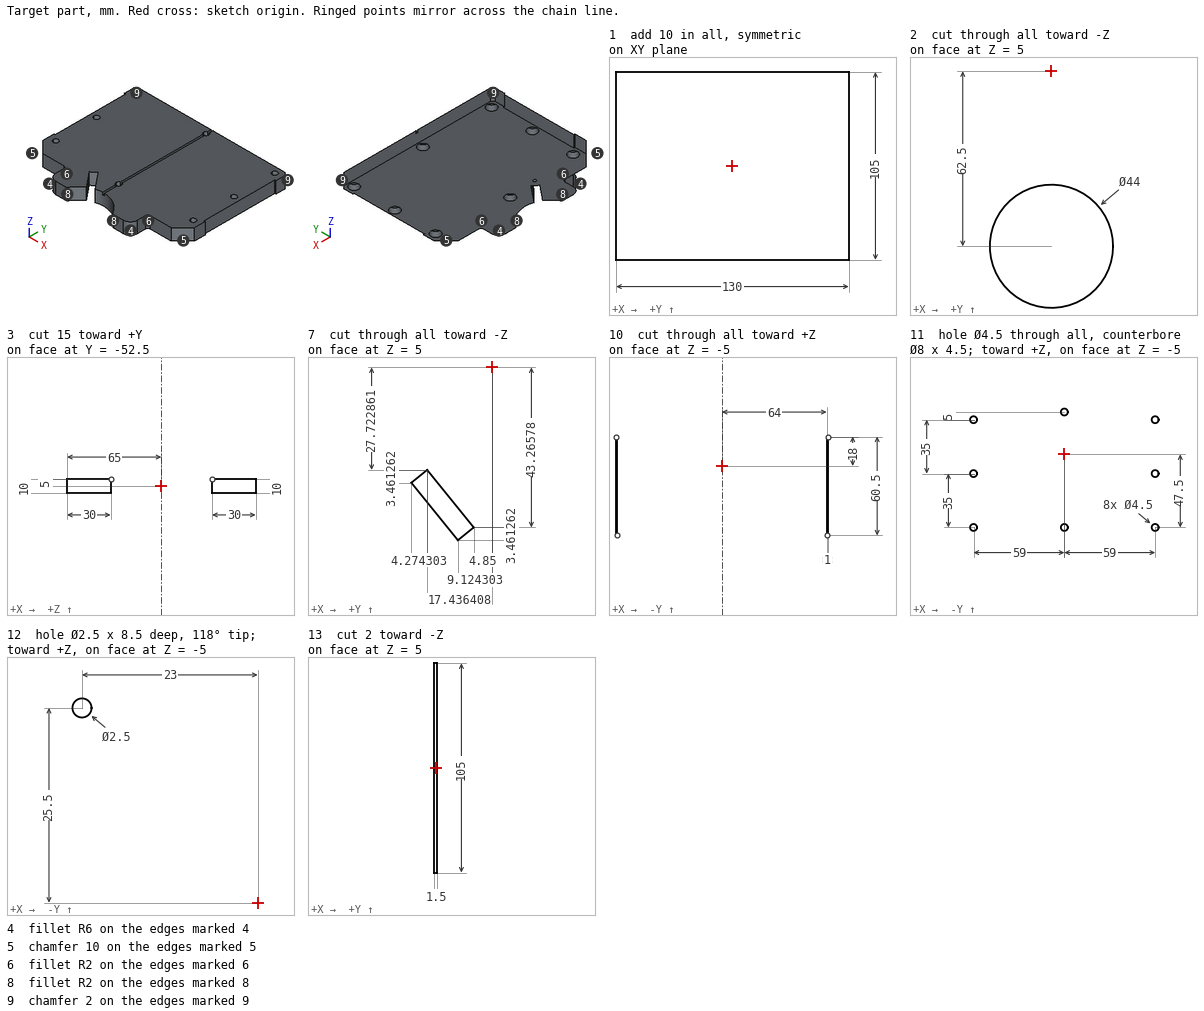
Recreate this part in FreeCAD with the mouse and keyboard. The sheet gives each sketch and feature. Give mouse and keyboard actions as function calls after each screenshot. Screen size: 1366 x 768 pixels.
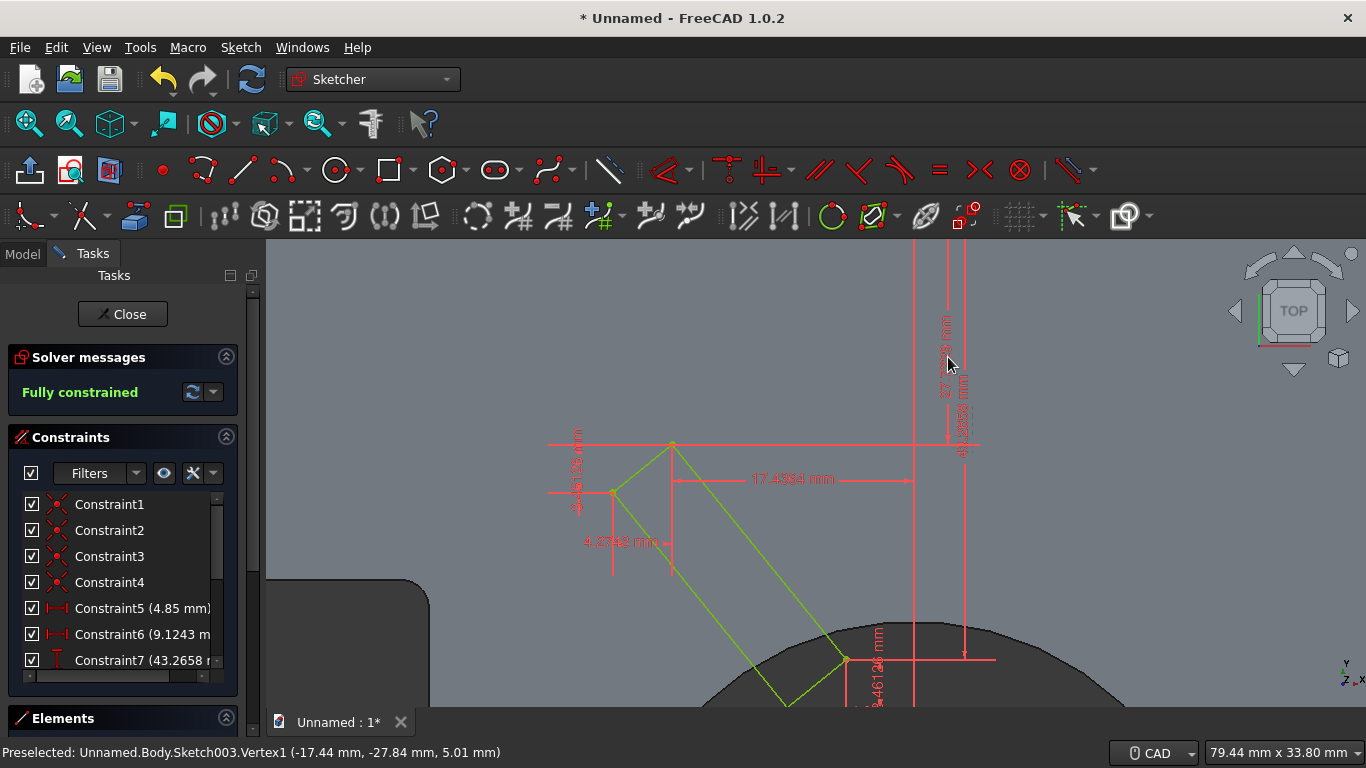
click(123, 314)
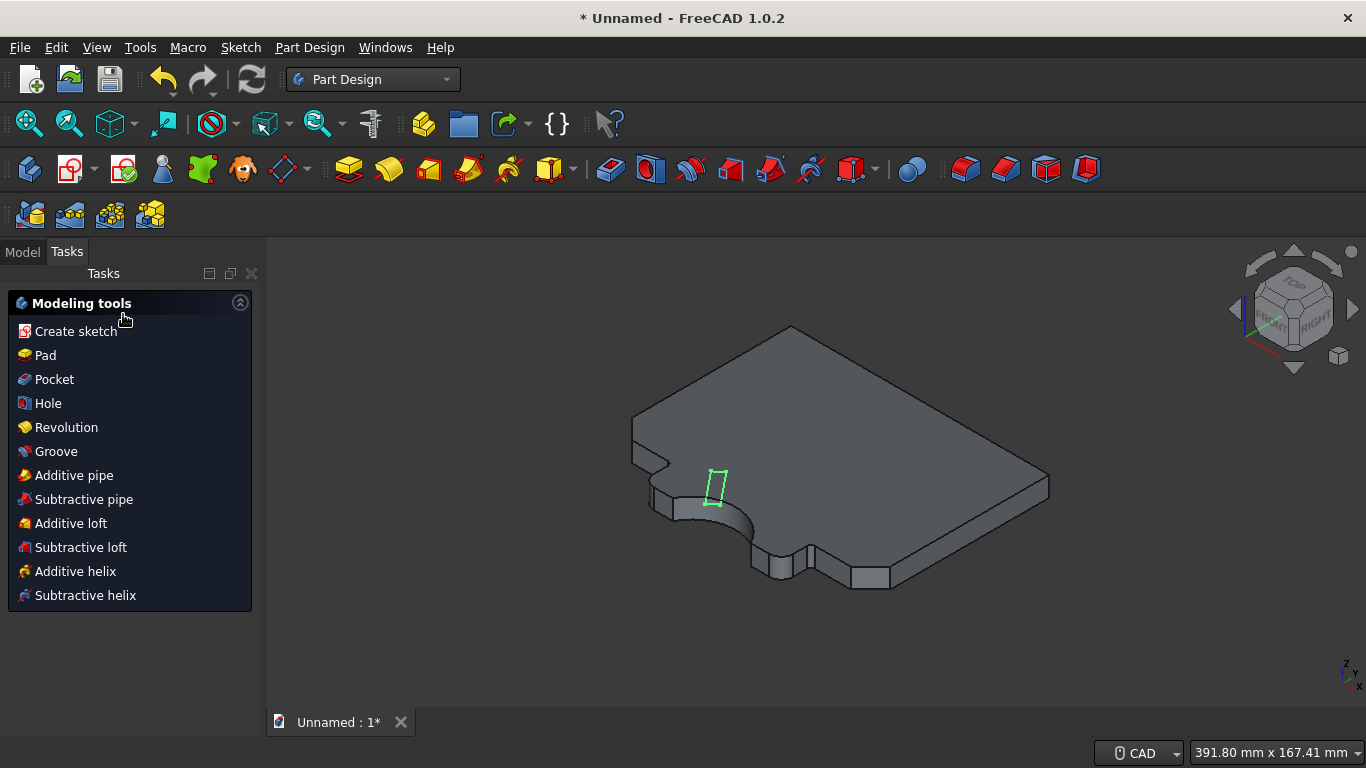
click(612, 170)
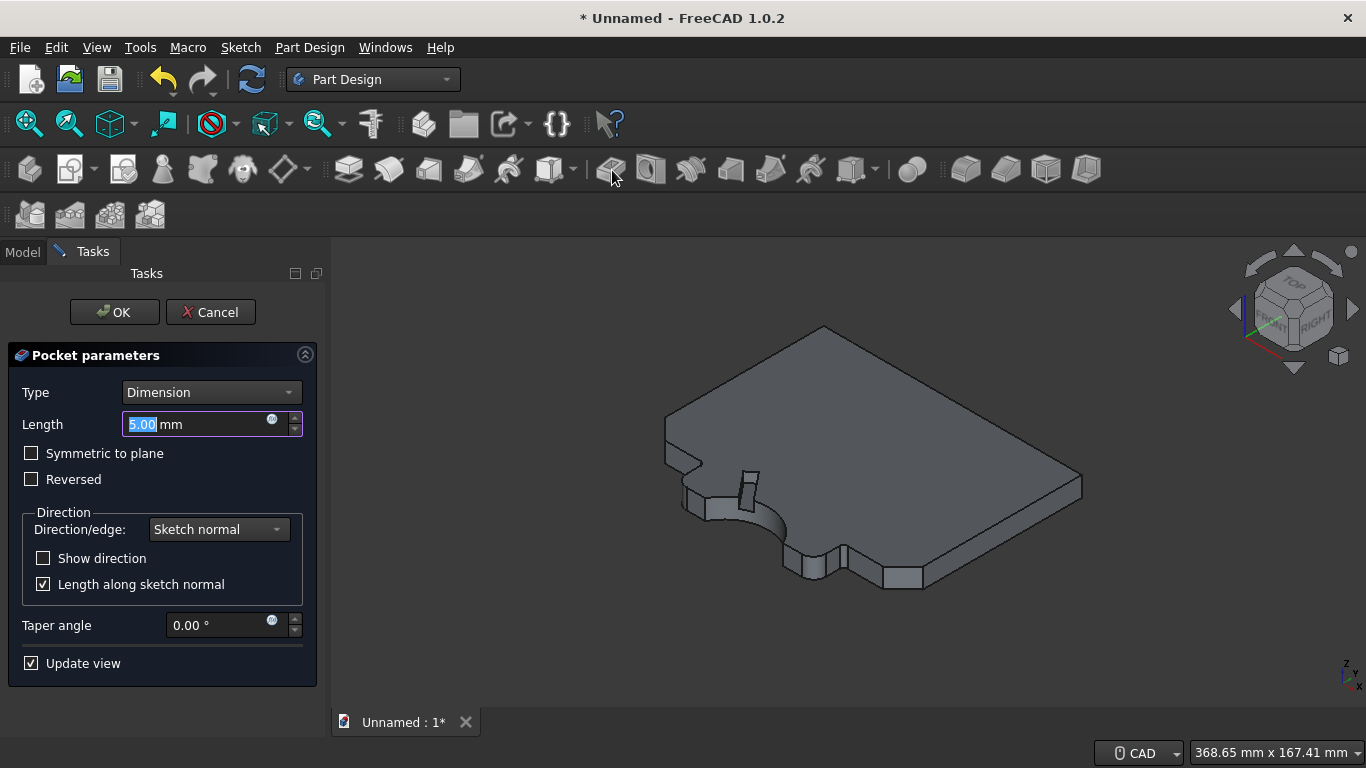
click(212, 392)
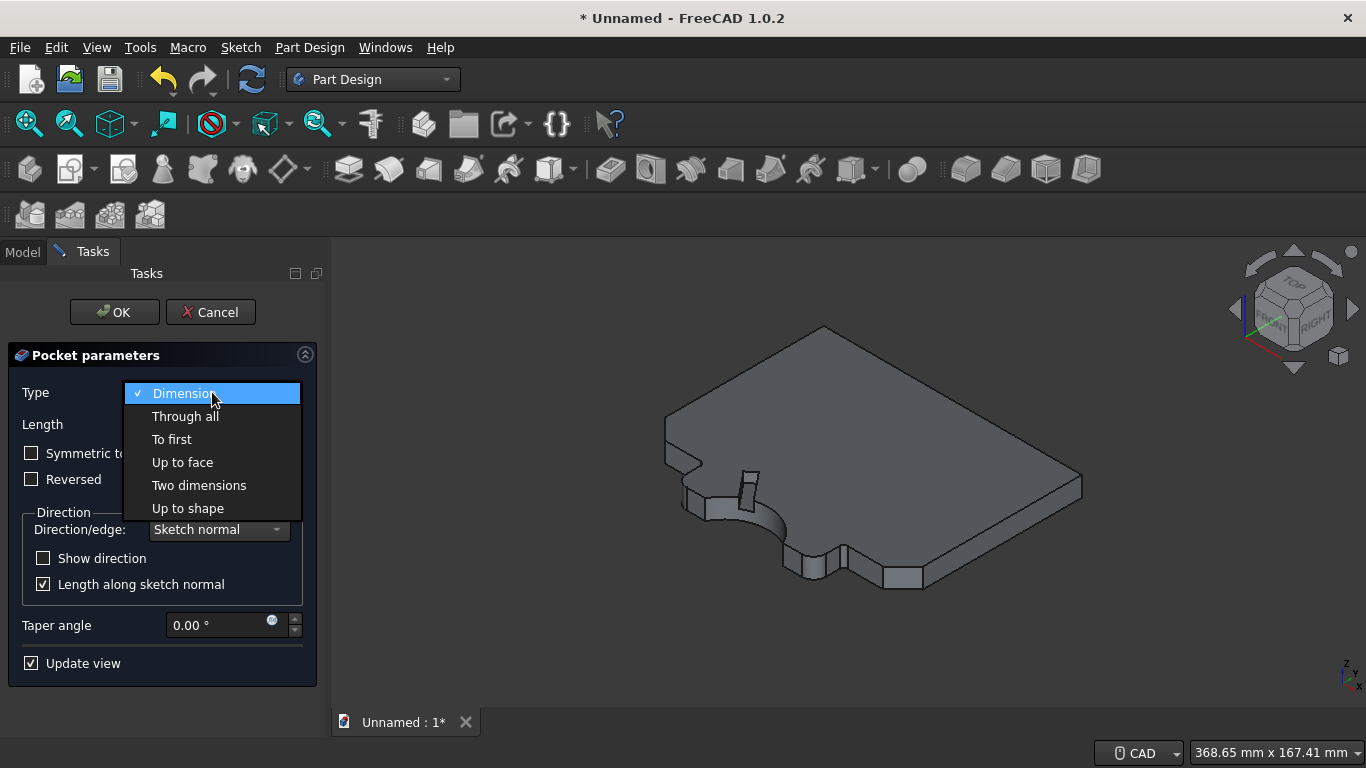
click(212, 416)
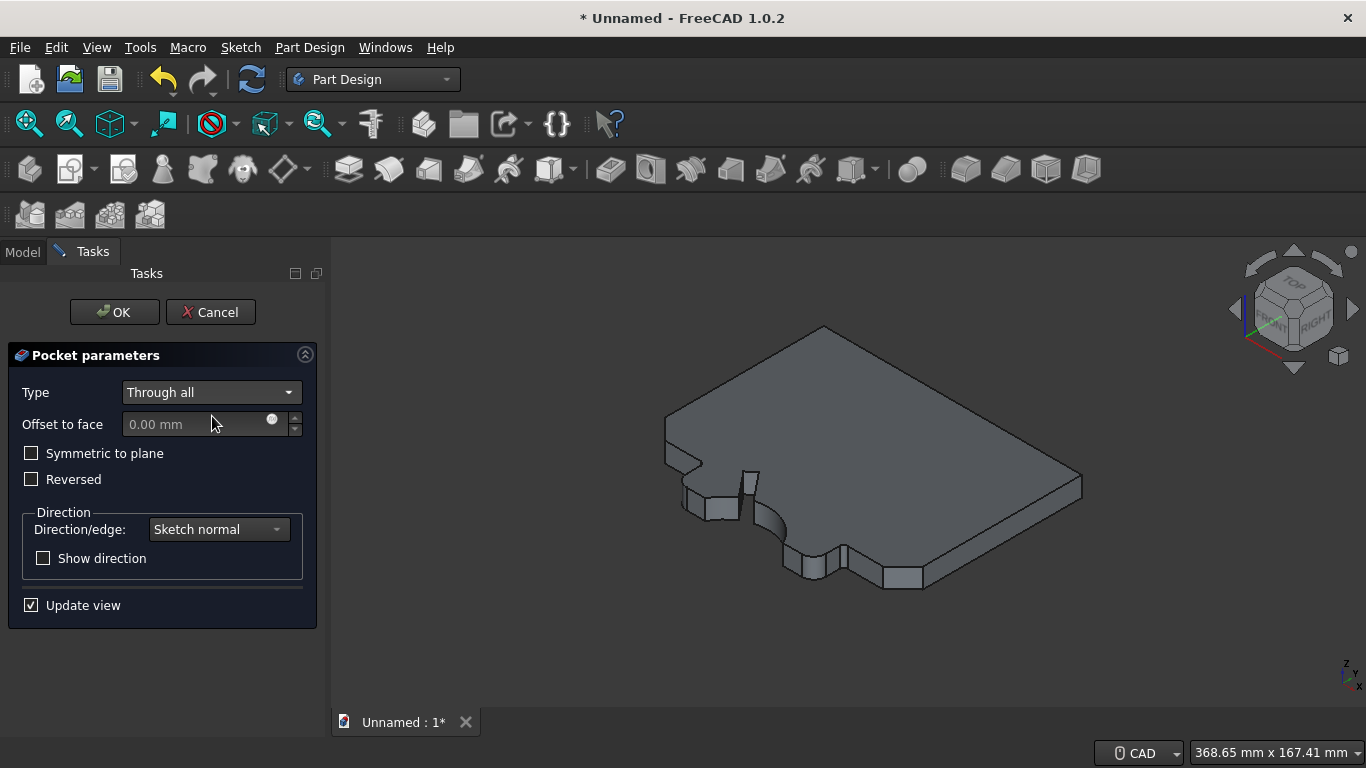
click(115, 312)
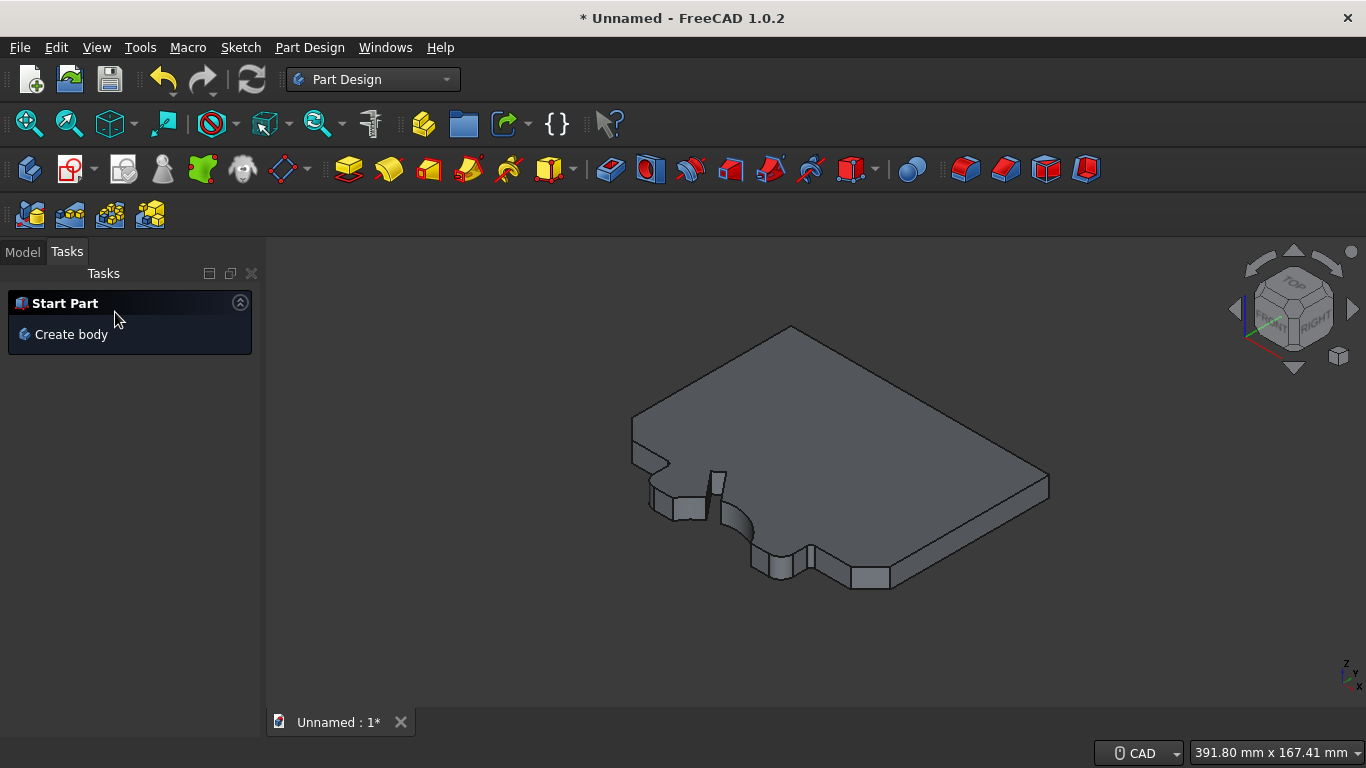
click(673, 509)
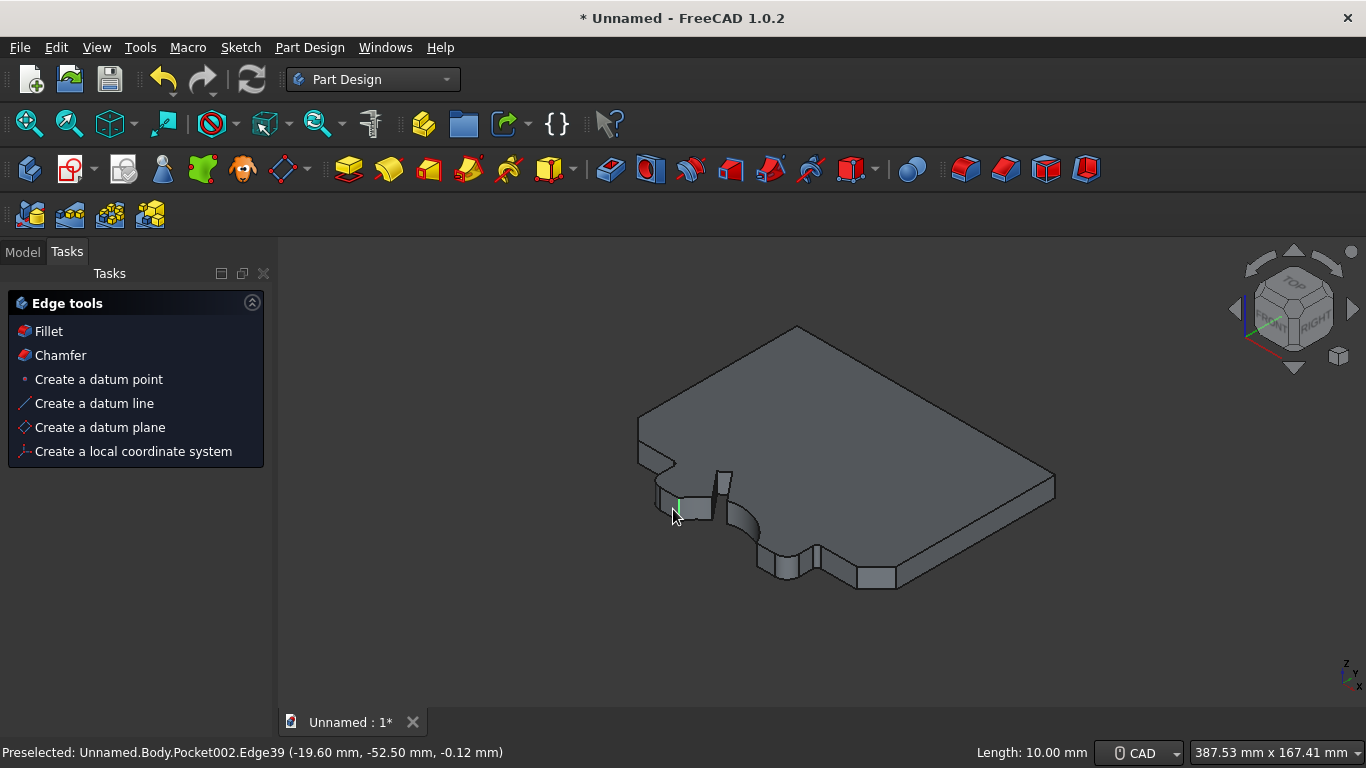
key(2)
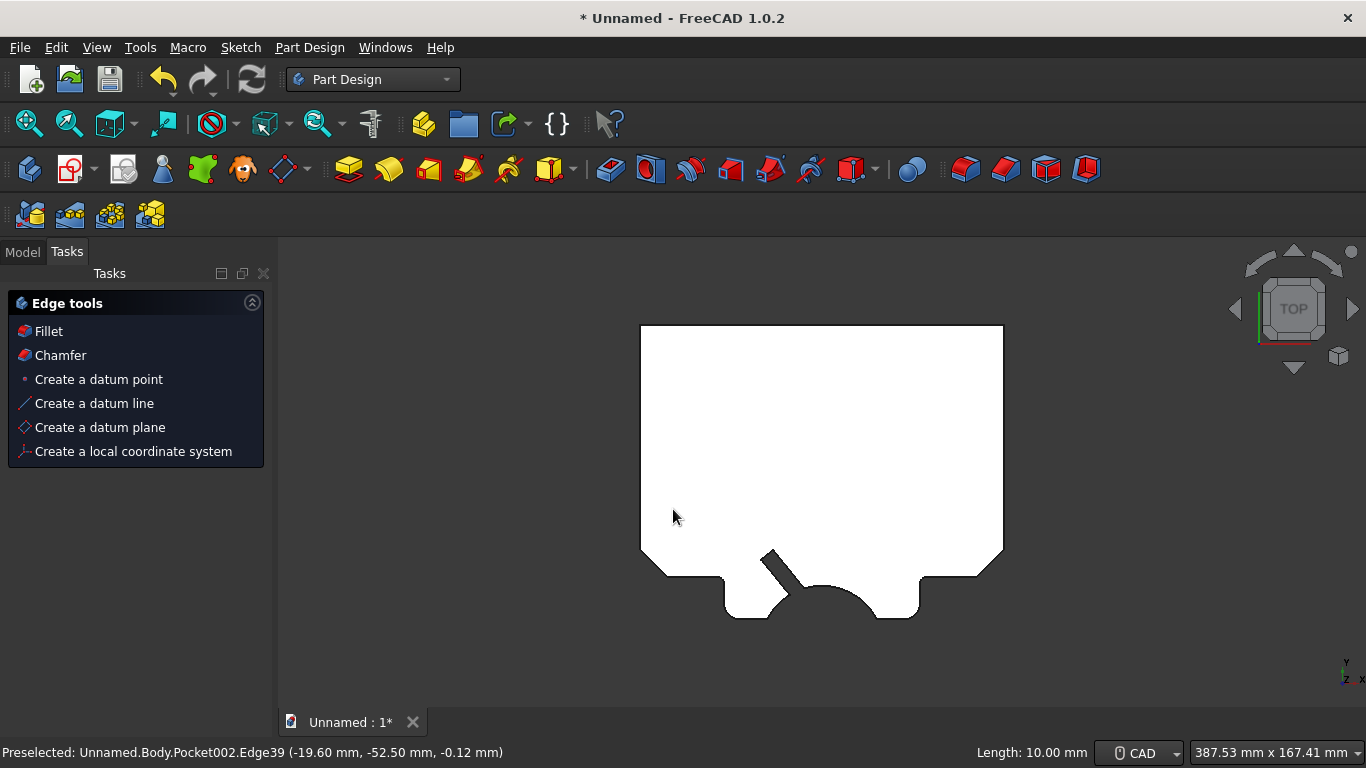
key(0)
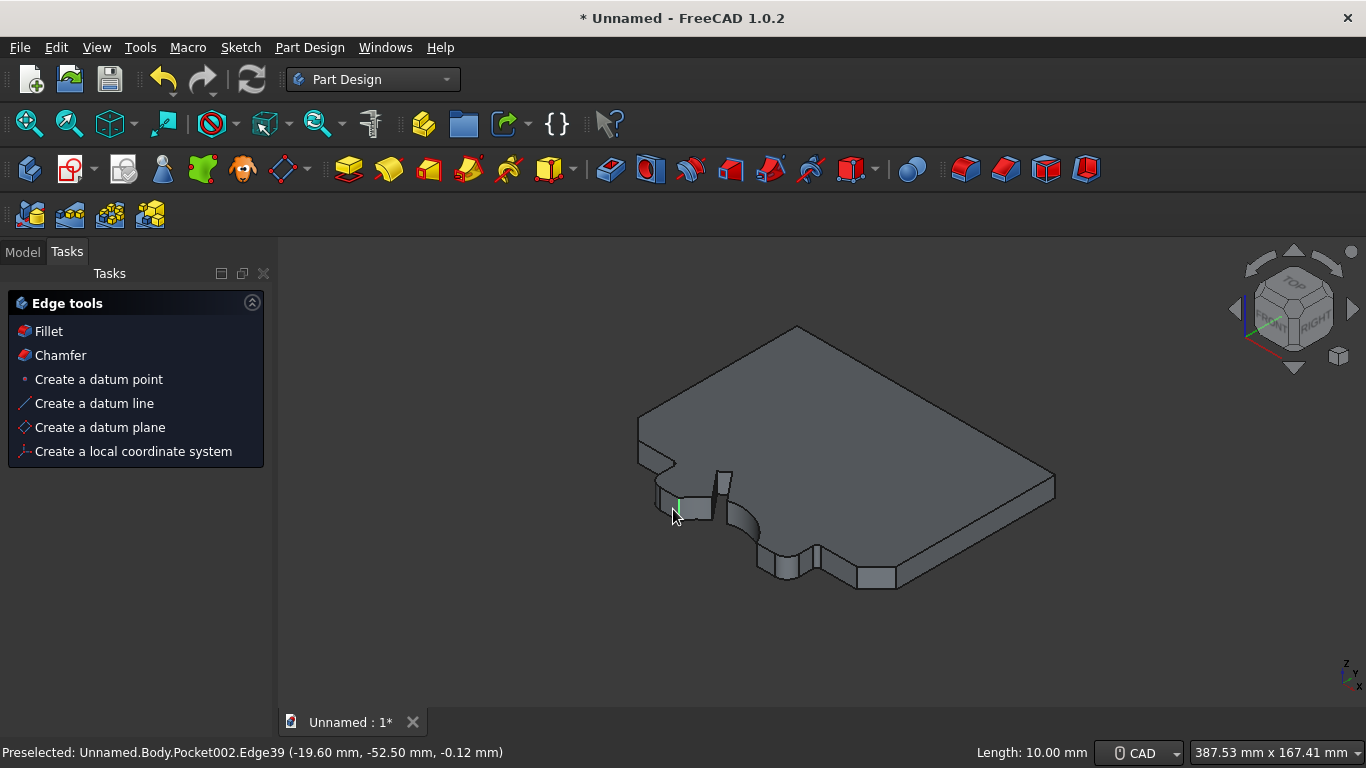
key(1)